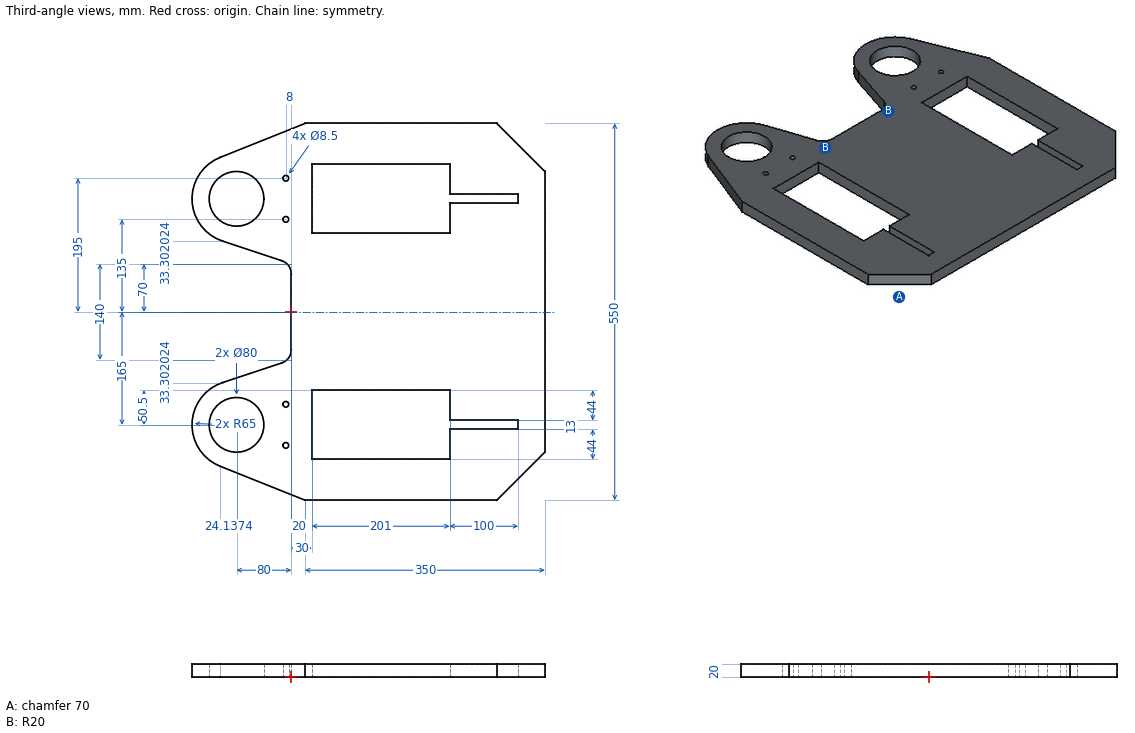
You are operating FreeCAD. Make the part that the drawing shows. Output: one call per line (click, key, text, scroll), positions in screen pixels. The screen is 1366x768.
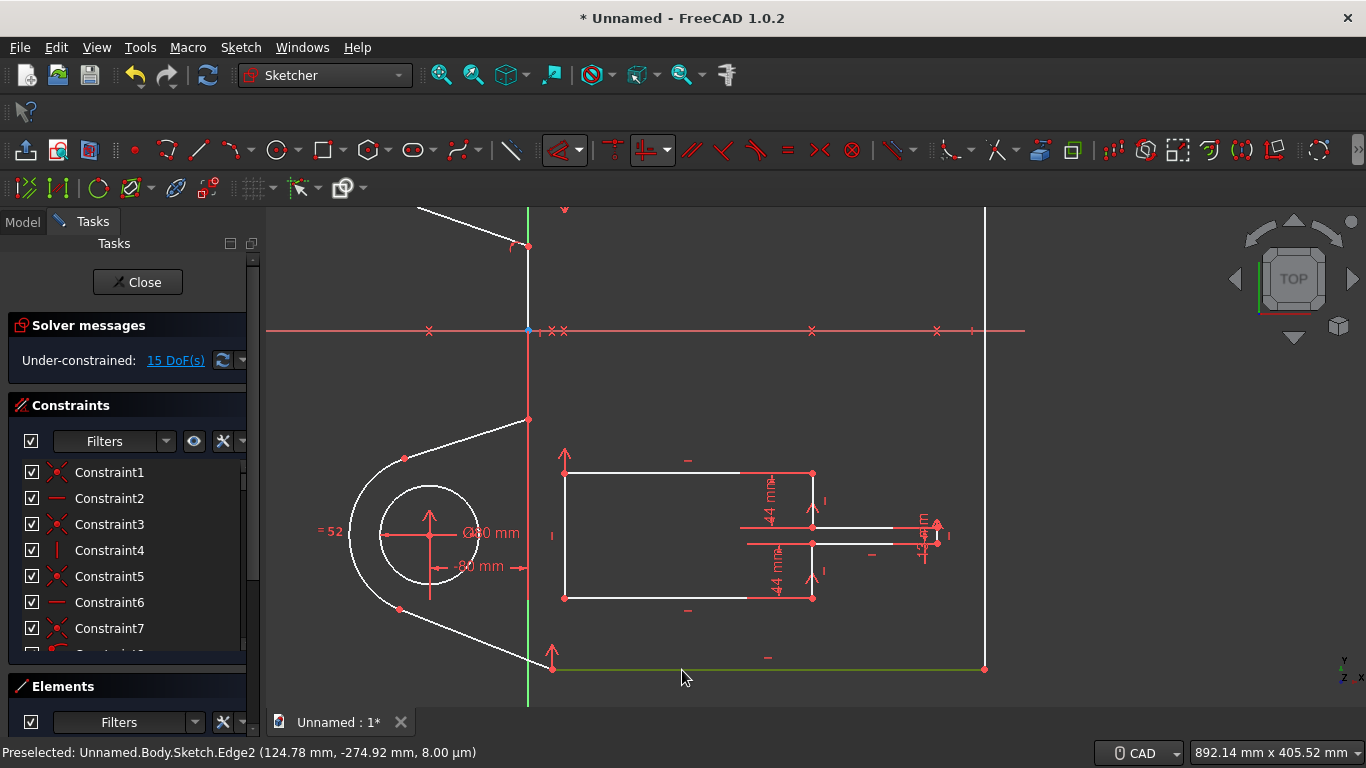
key(l)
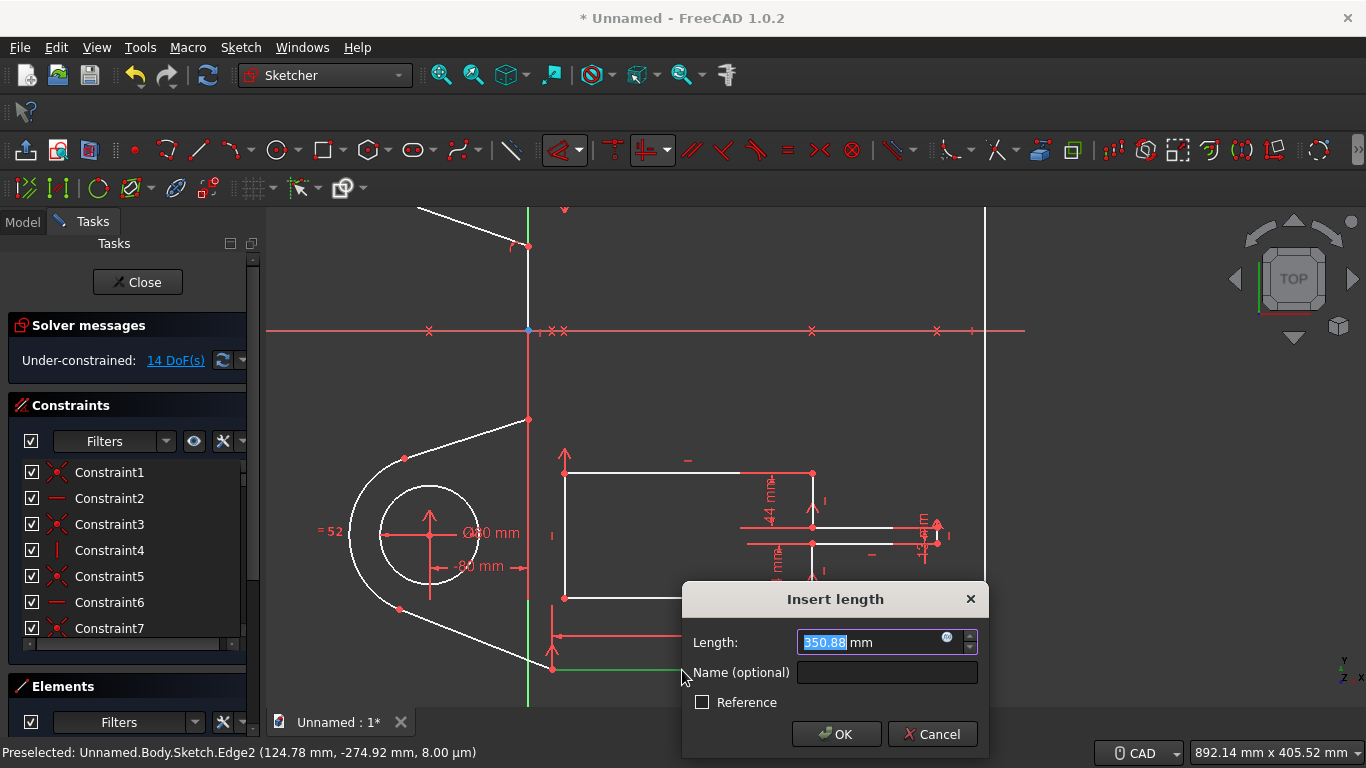
text(350)
key(Return)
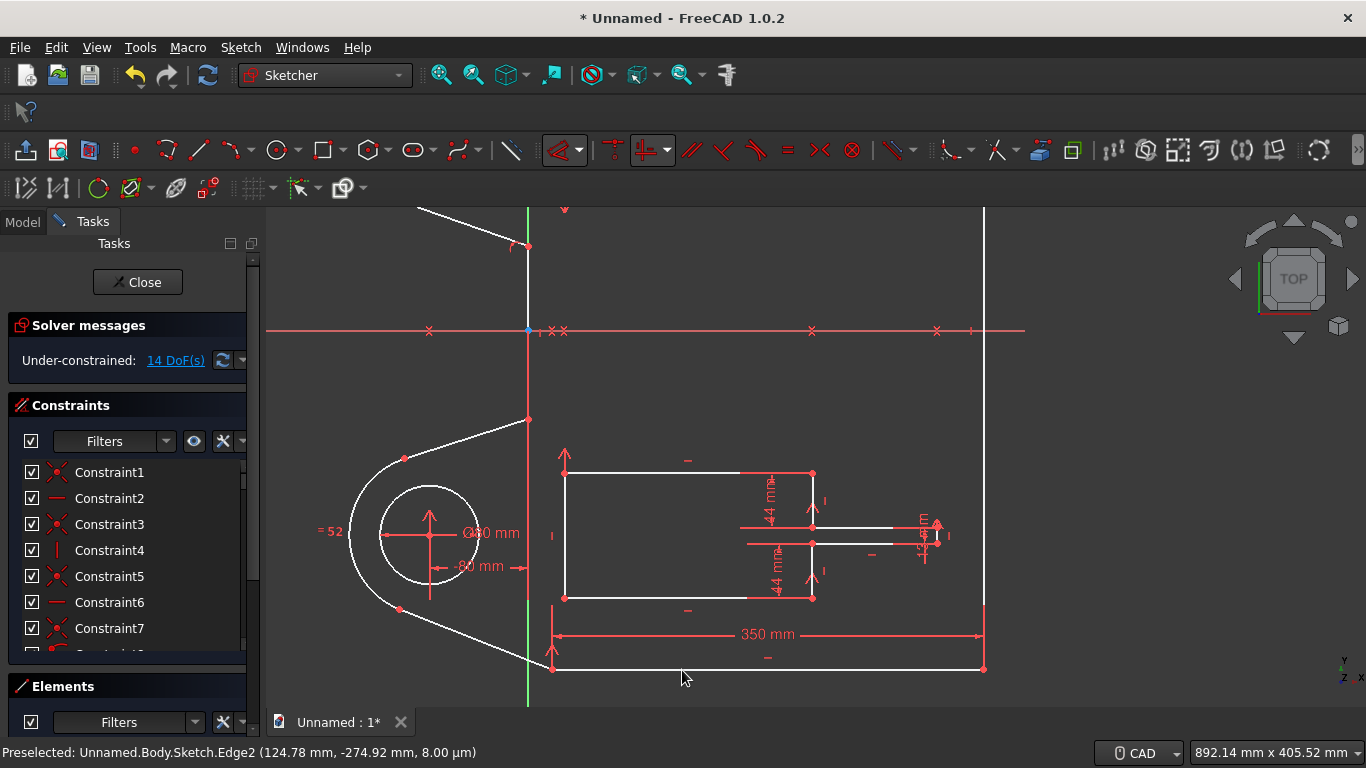
click(984, 466)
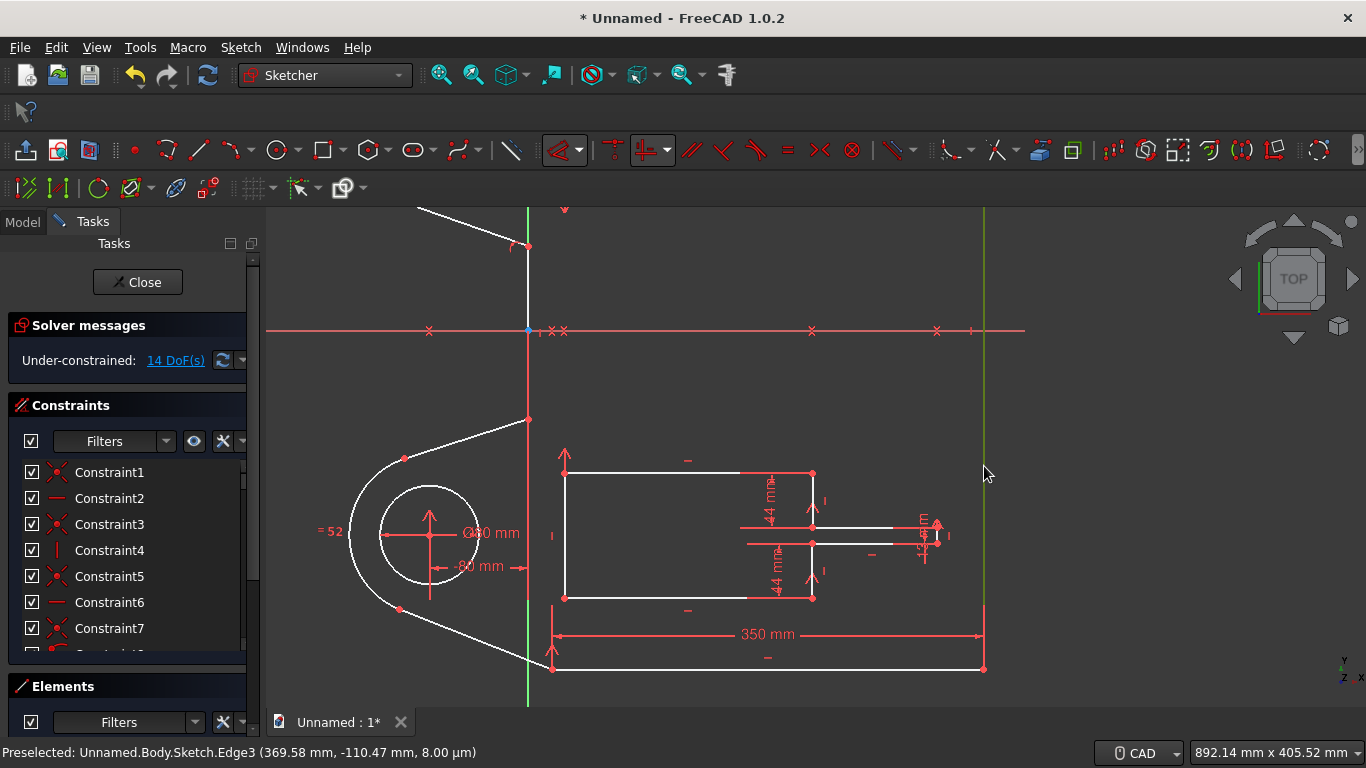
key(i)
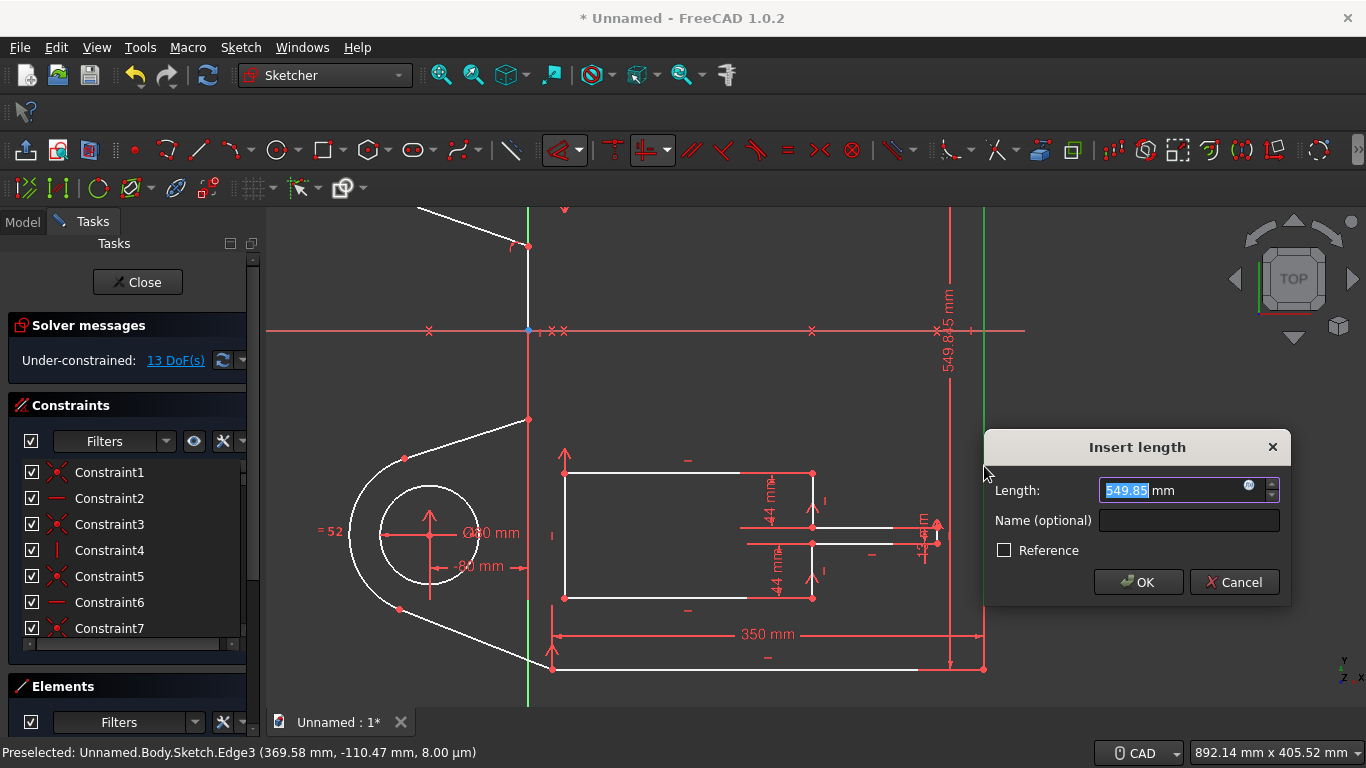
text(550)
key(Return)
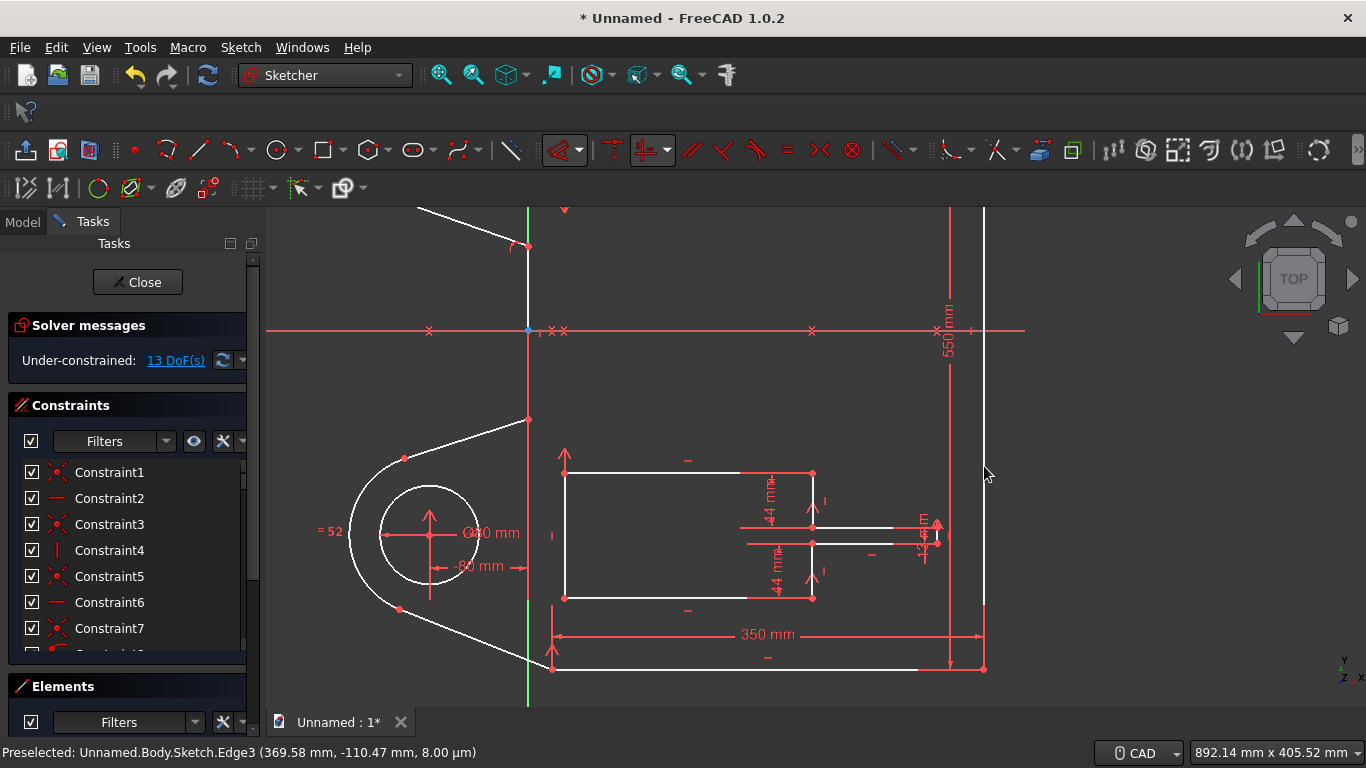
click(528, 298)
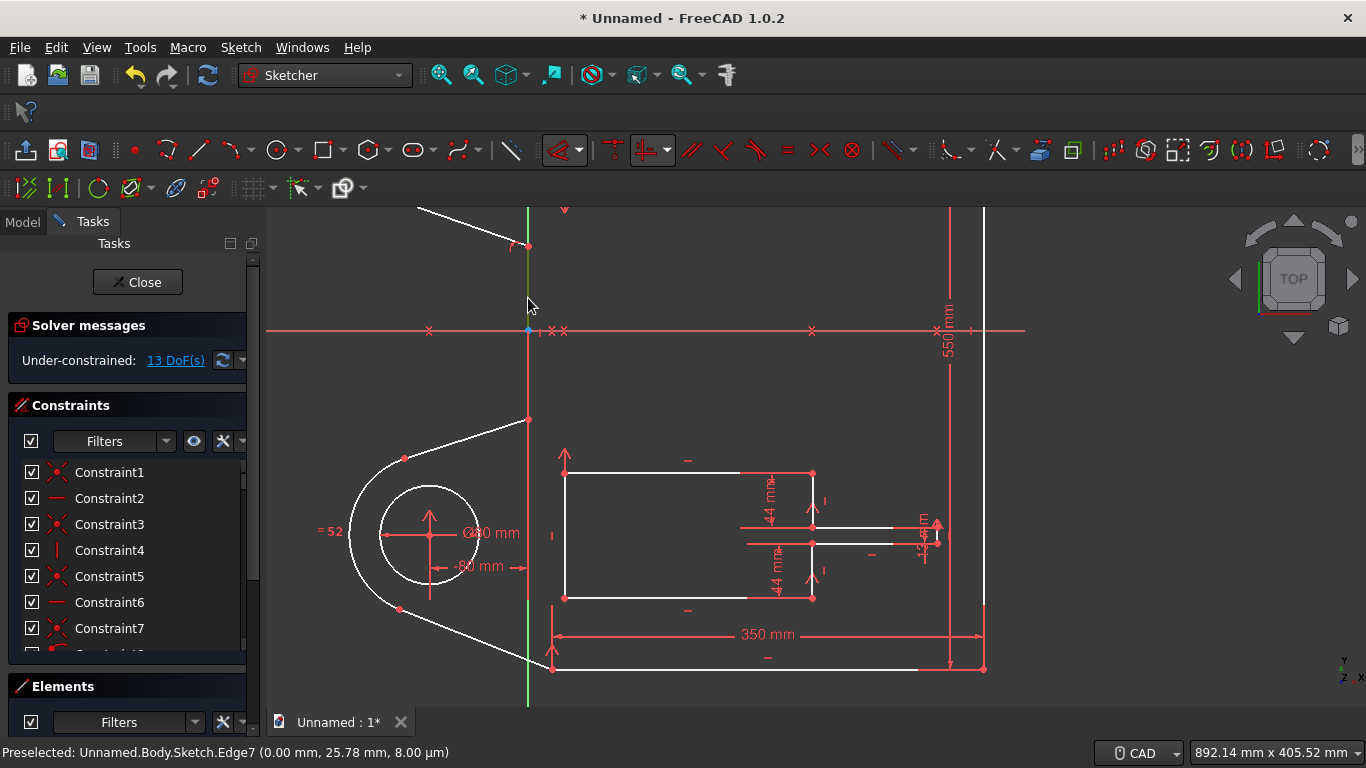
key(i)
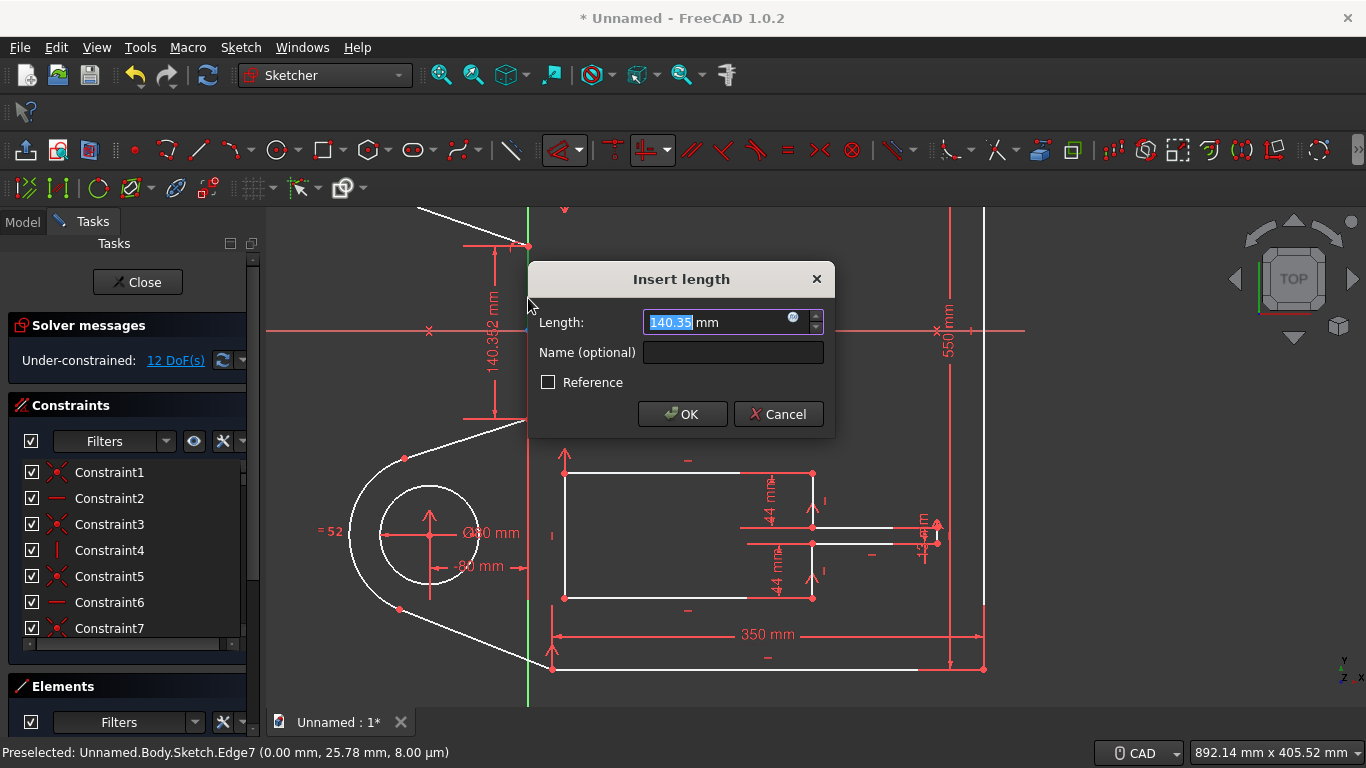
text(140)
key(Return)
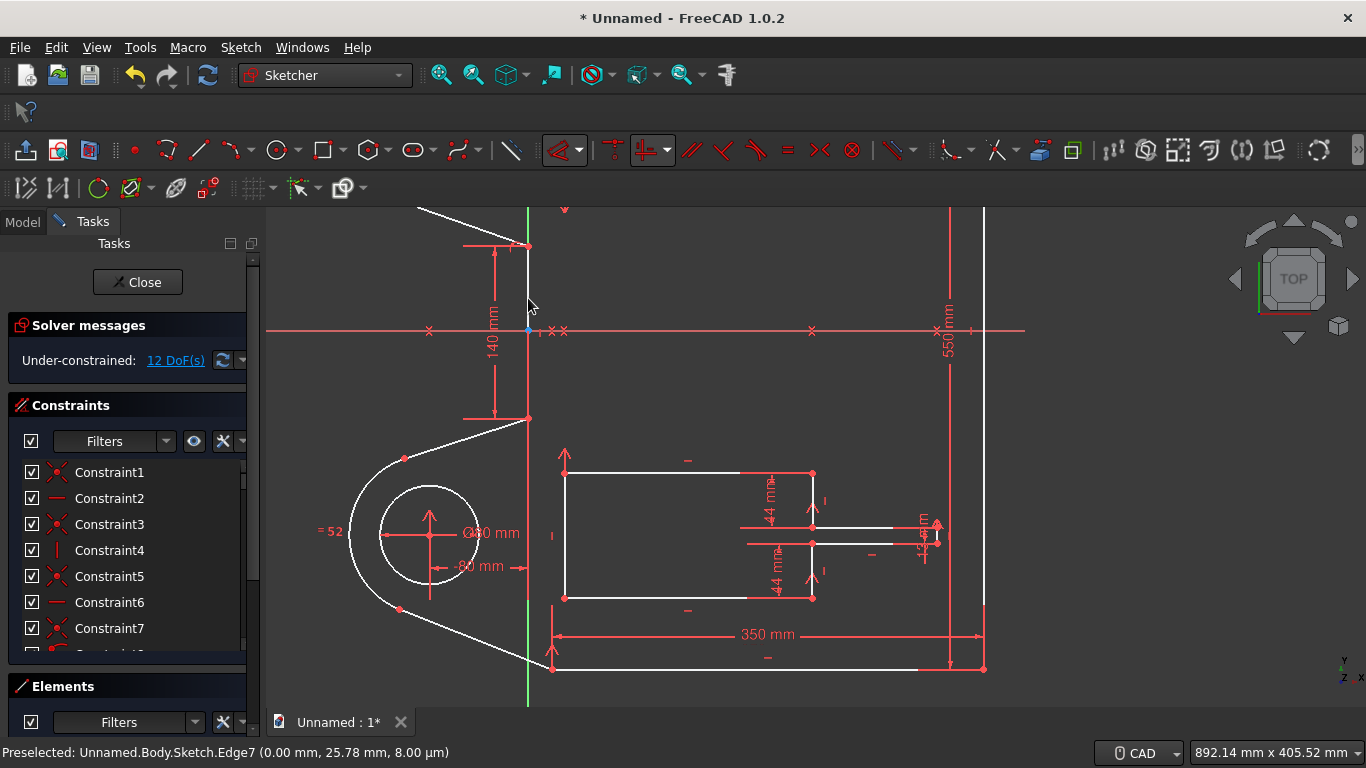
click(639, 473)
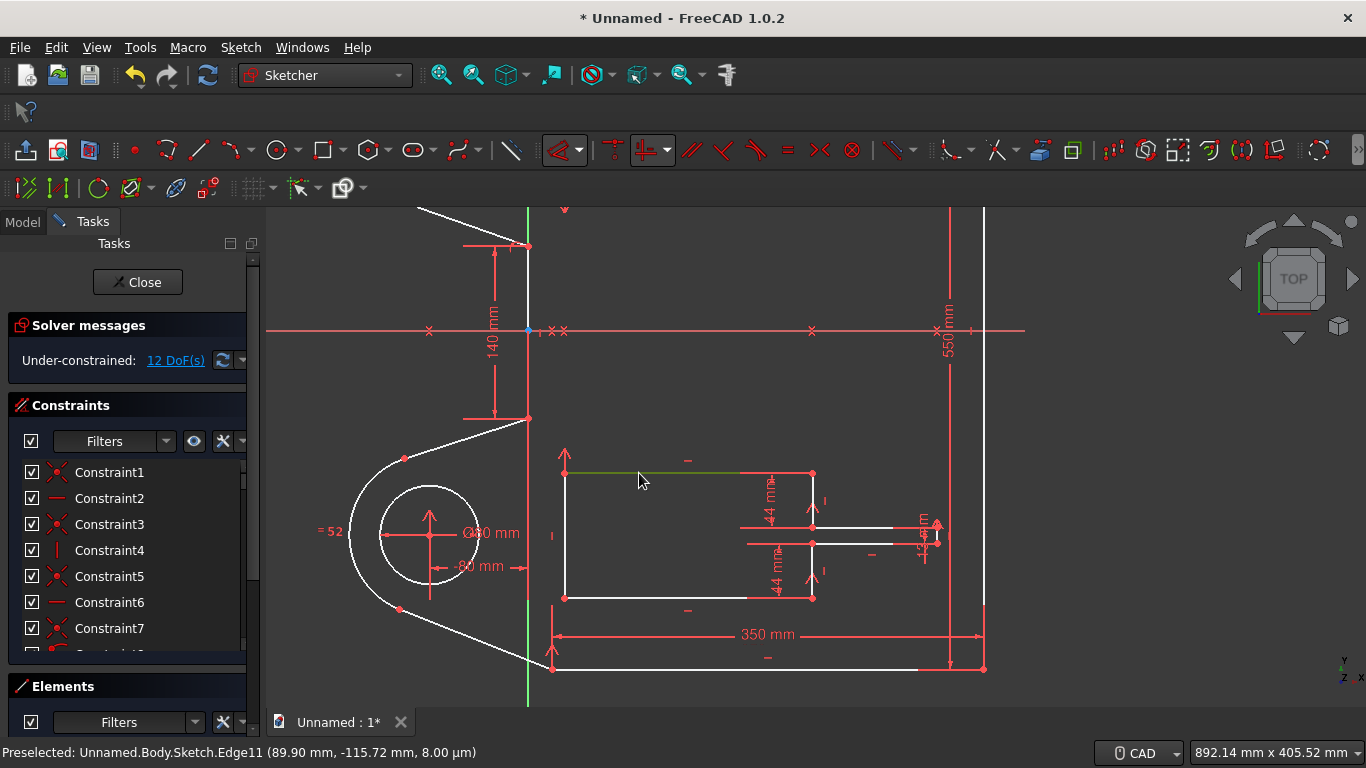
key(l)